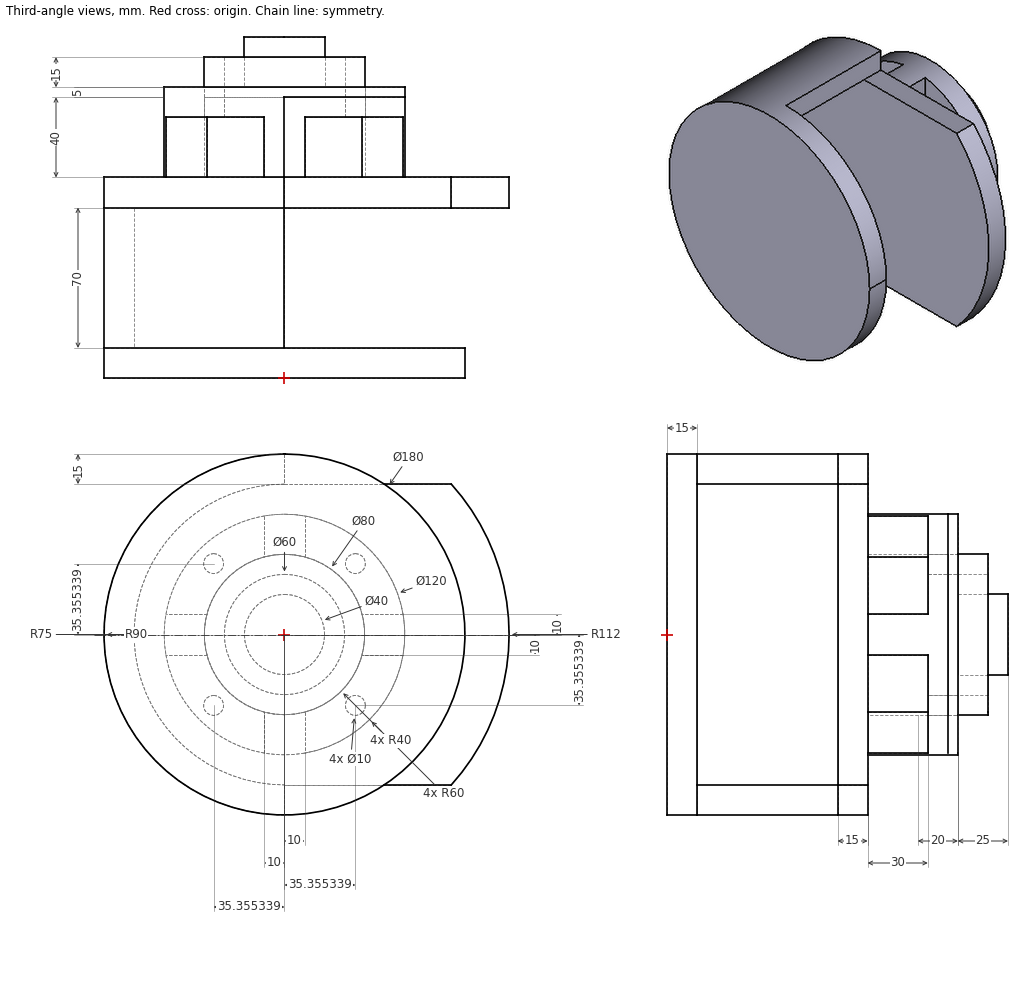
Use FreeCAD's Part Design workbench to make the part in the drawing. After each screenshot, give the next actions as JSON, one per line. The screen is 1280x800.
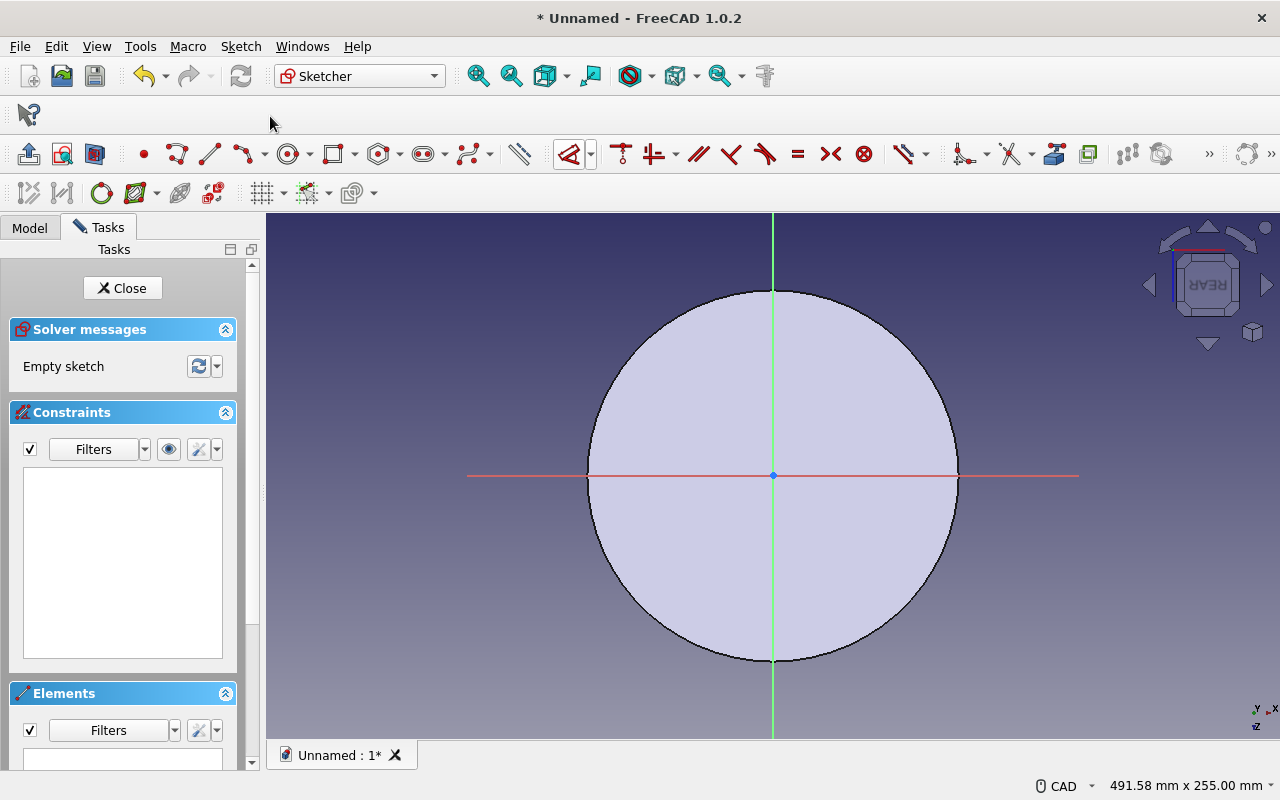
{"action": "left_click", "coordinate": [210, 154]}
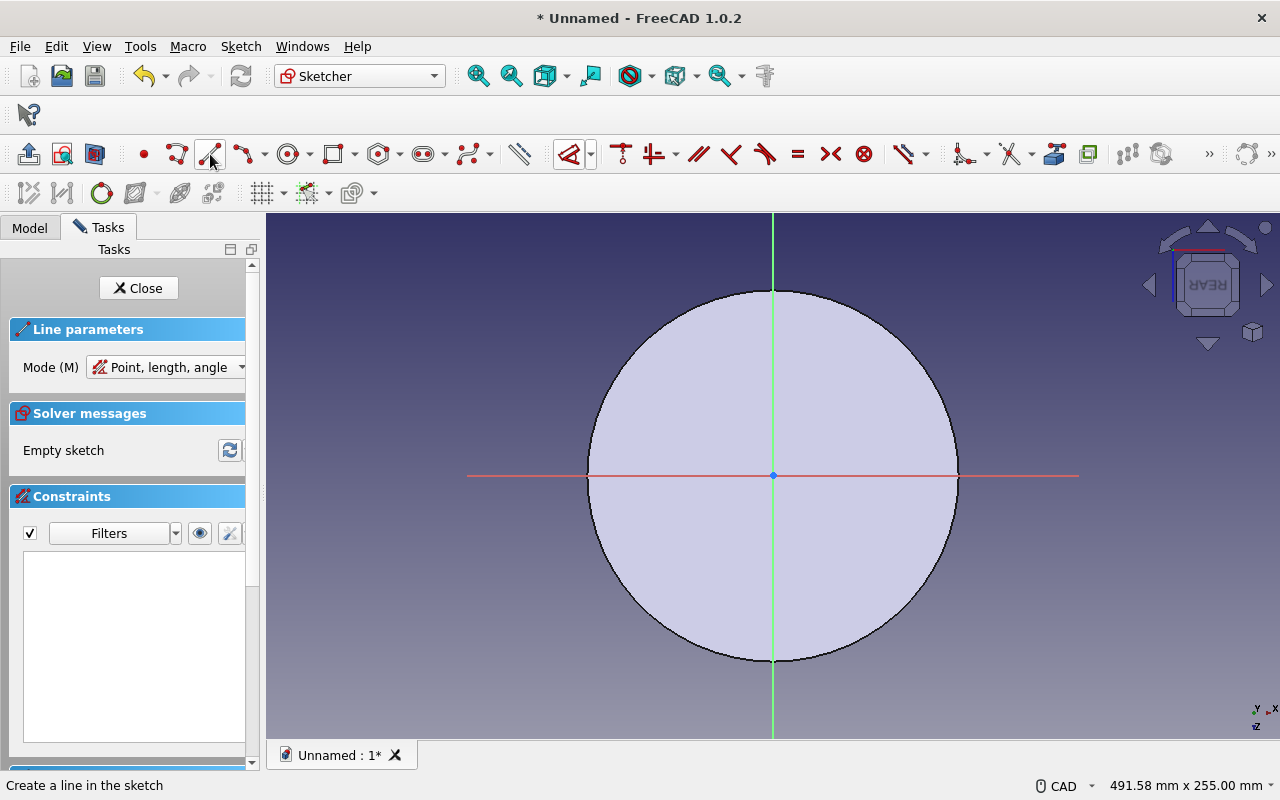
{"action": "left_click", "coordinate": [773, 662]}
{"action": "left_click", "coordinate": [764, 631]}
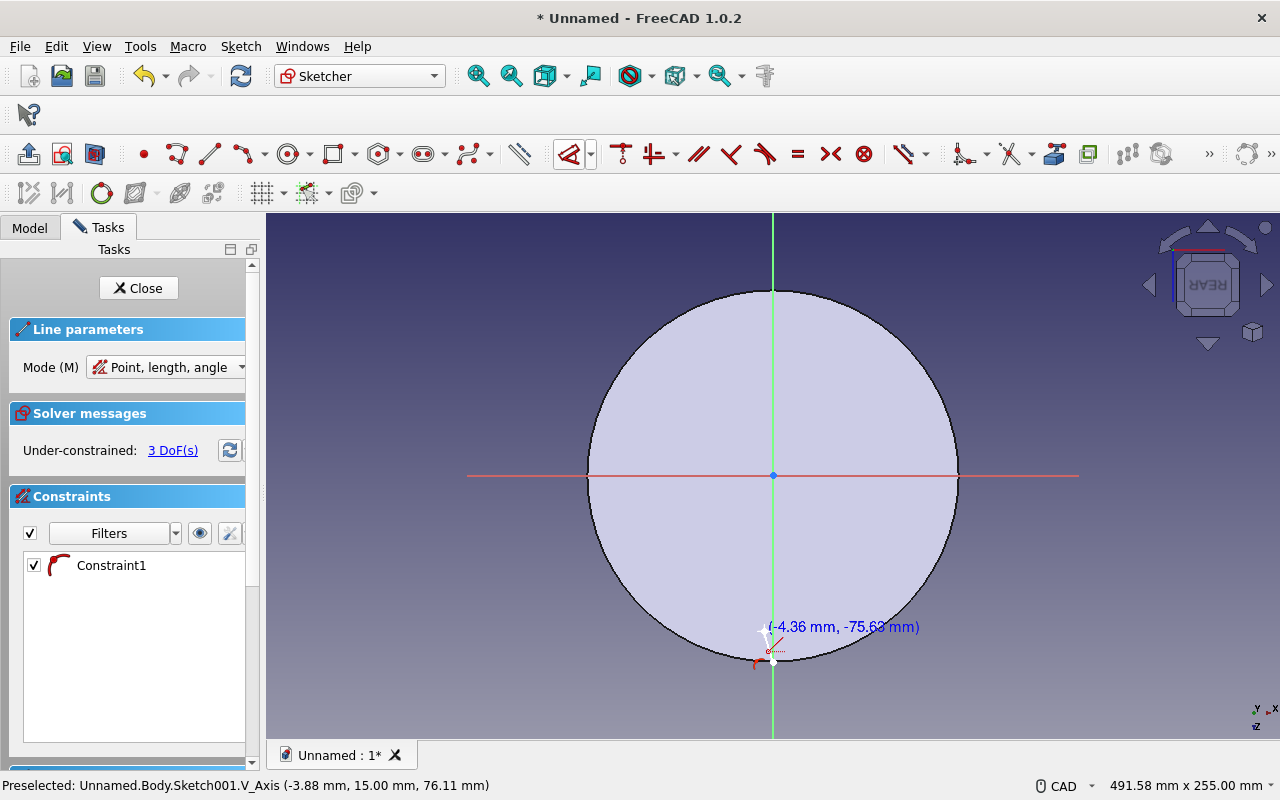
{"action": "left_click", "coordinate": [773, 321]}
{"action": "left_click", "coordinate": [764, 290]}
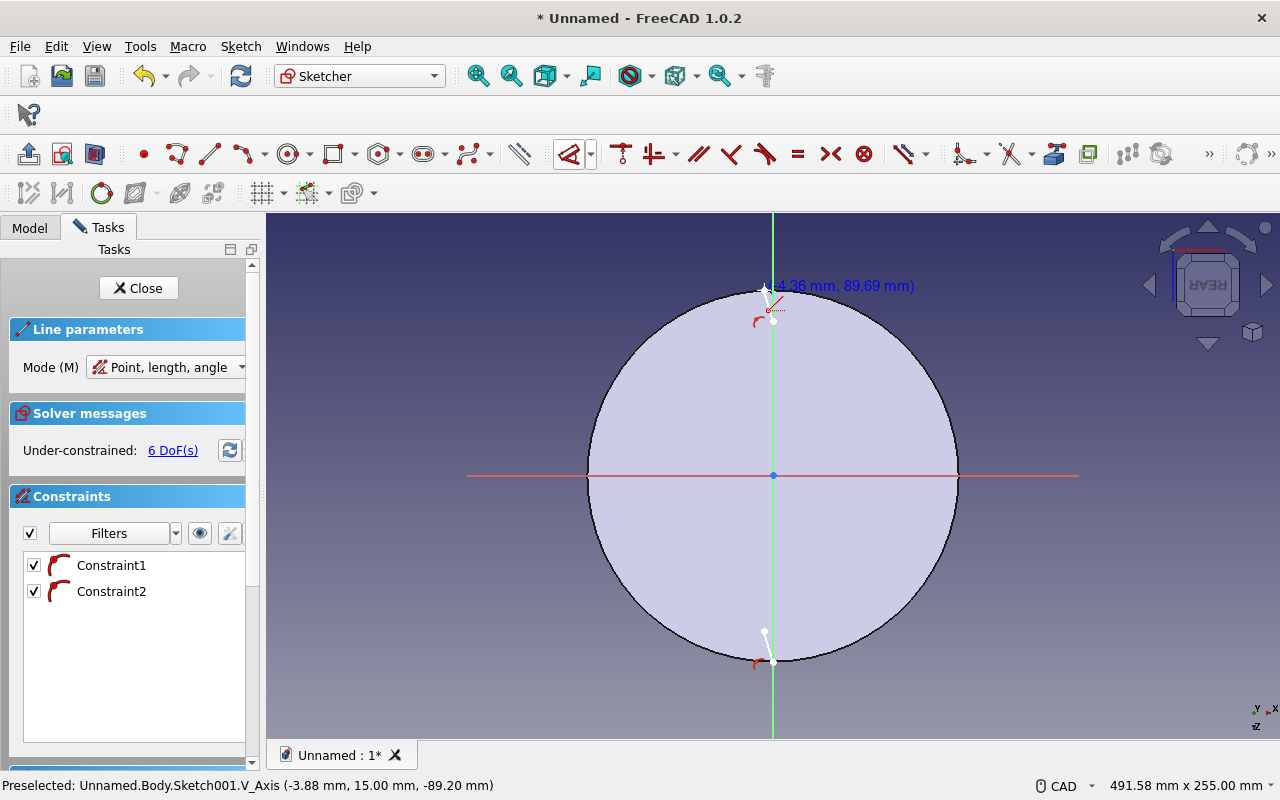
{"action": "left_click", "coordinate": [242, 154]}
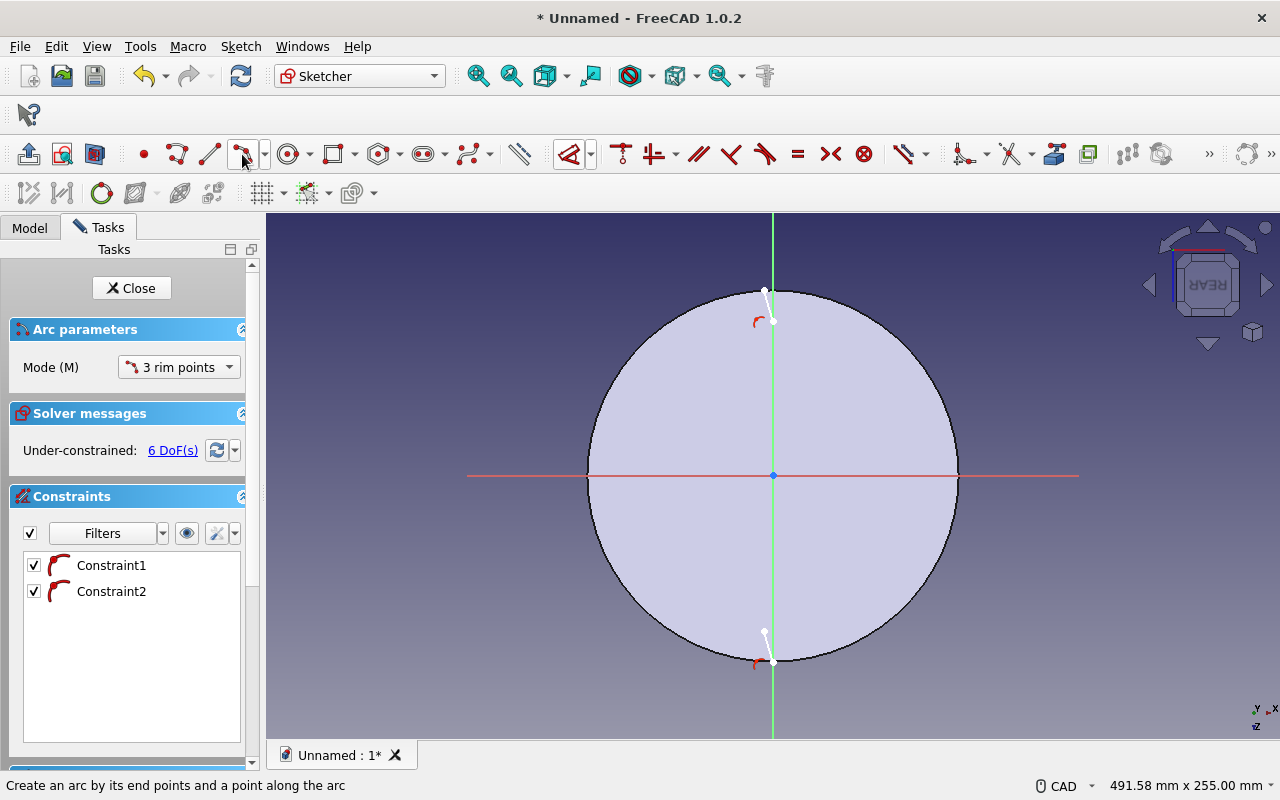
{"action": "left_click", "coordinate": [764, 632]}
{"action": "left_click", "coordinate": [773, 322]}
{"action": "left_click", "coordinate": [626, 428]}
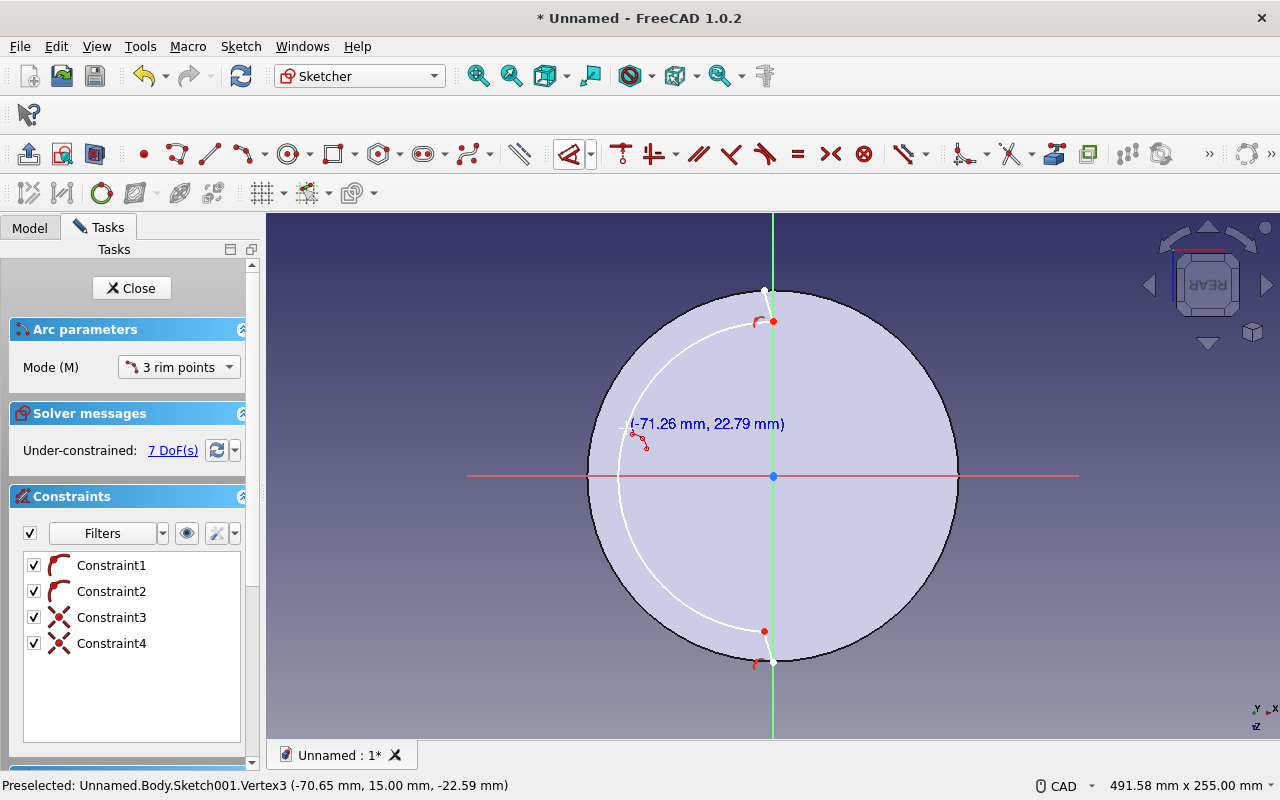
{"action": "left_click", "coordinate": [764, 291]}
{"action": "left_click", "coordinate": [773, 663]}
{"action": "left_click", "coordinate": [596, 419]}
{"action": "key", "text": "Escape"}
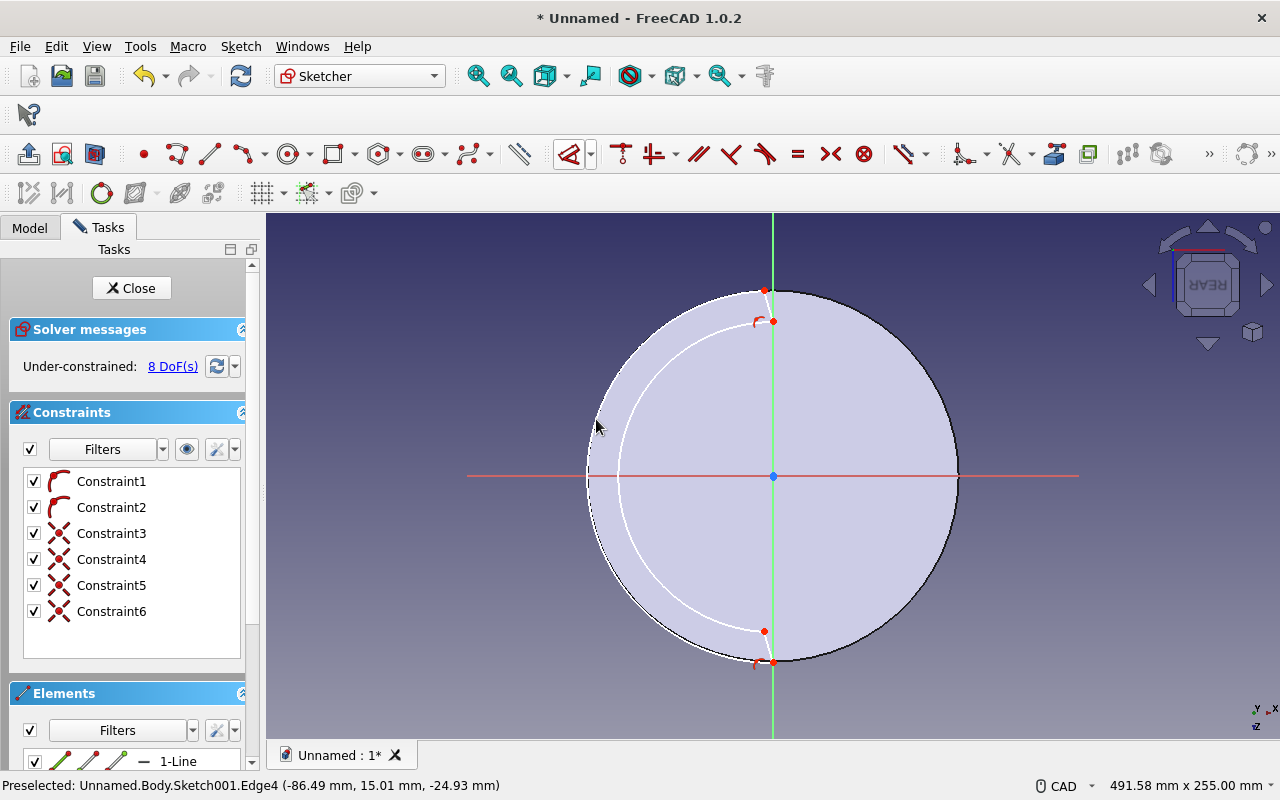
{"action": "scroll", "coordinate": [770, 654], "scroll_direction": "up", "scroll_amount": 2}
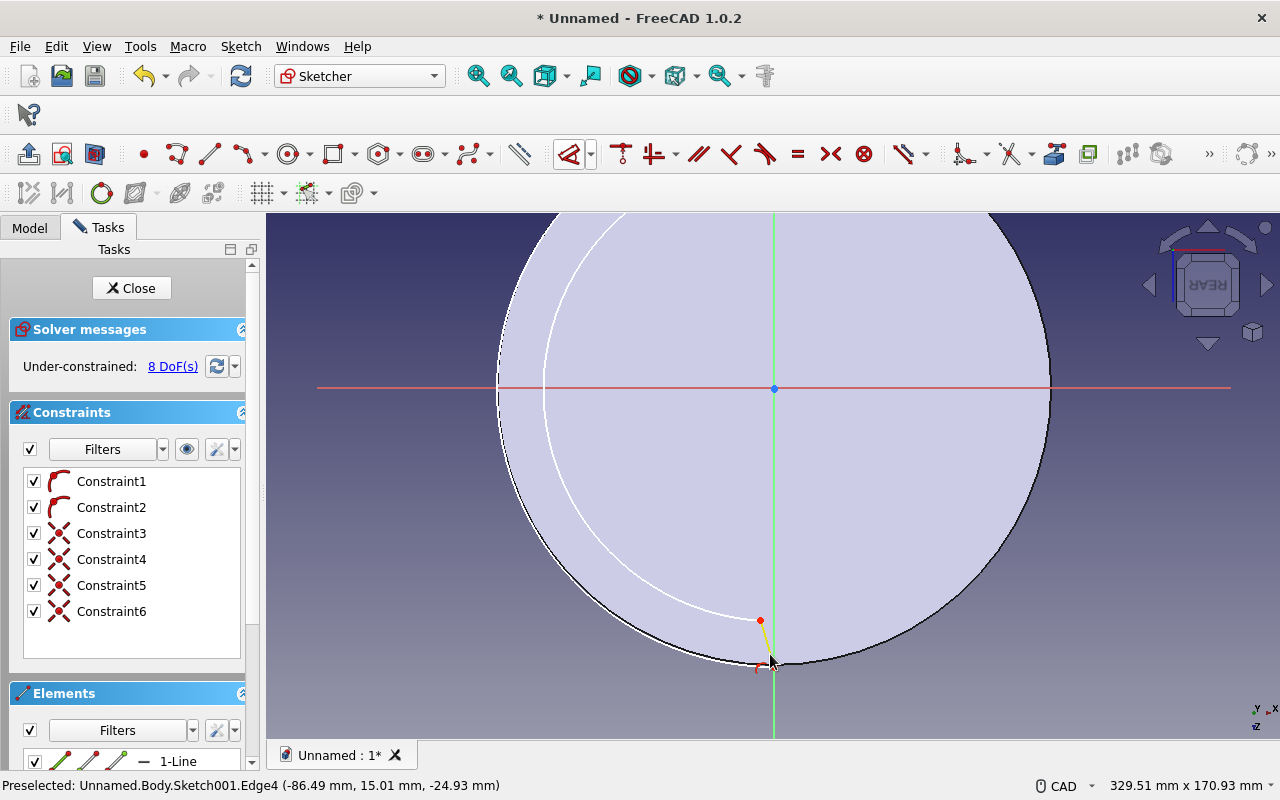
{"action": "left_click", "coordinate": [770, 653]}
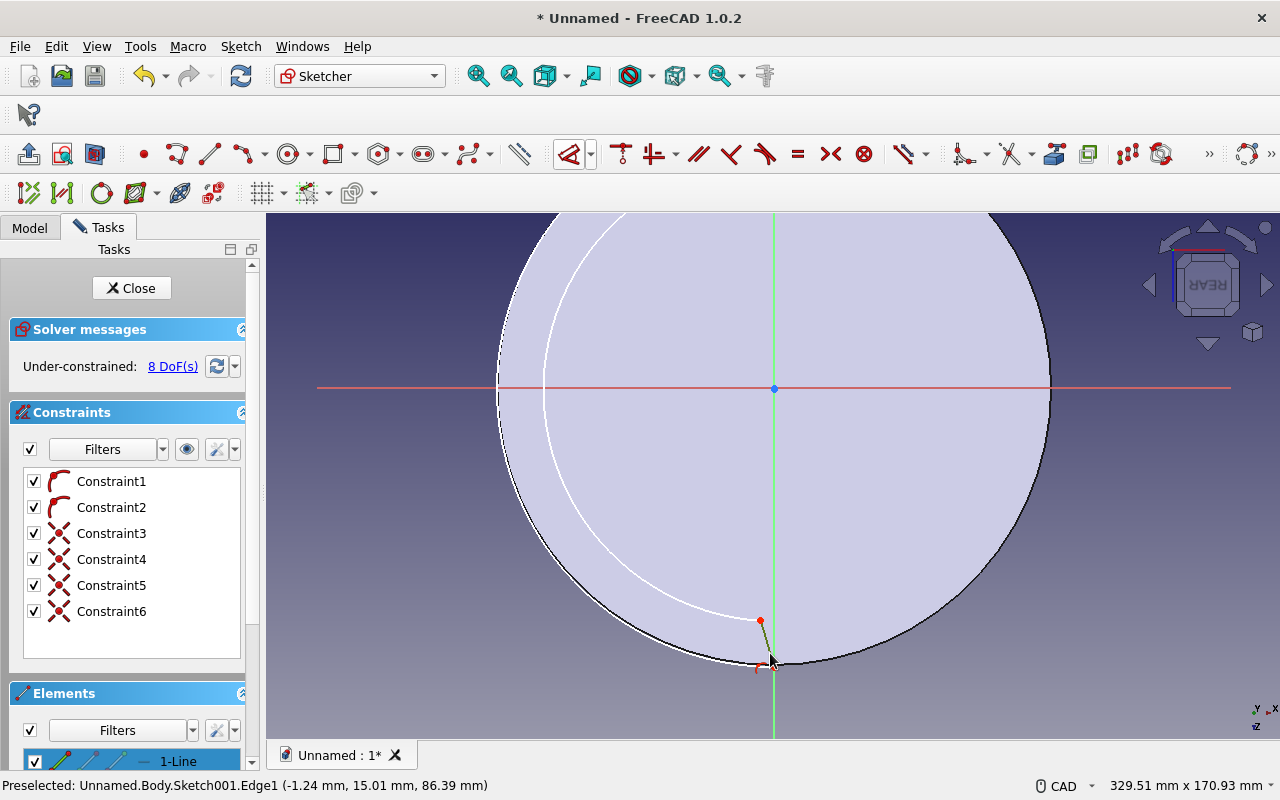
{"action": "key", "text": "v"}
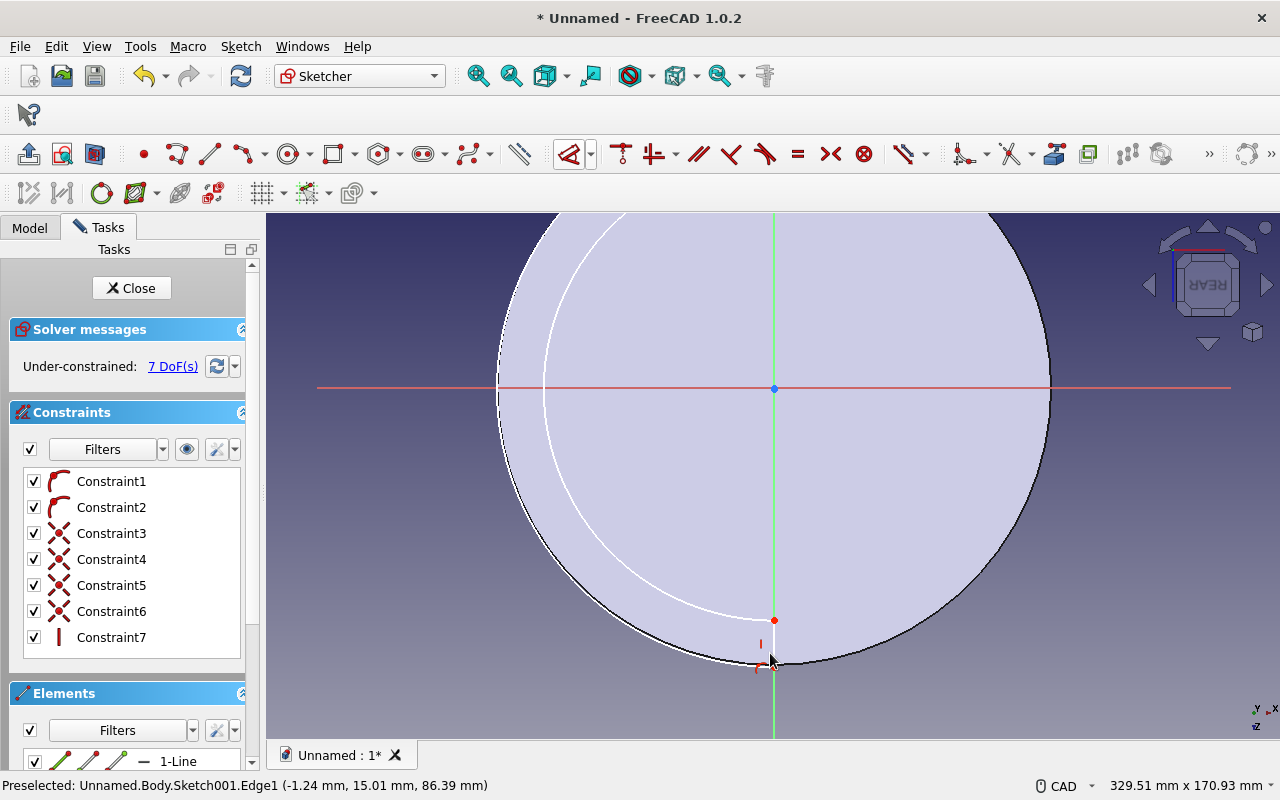
{"action": "scroll", "coordinate": [788, 583], "scroll_direction": "down", "scroll_amount": 3}